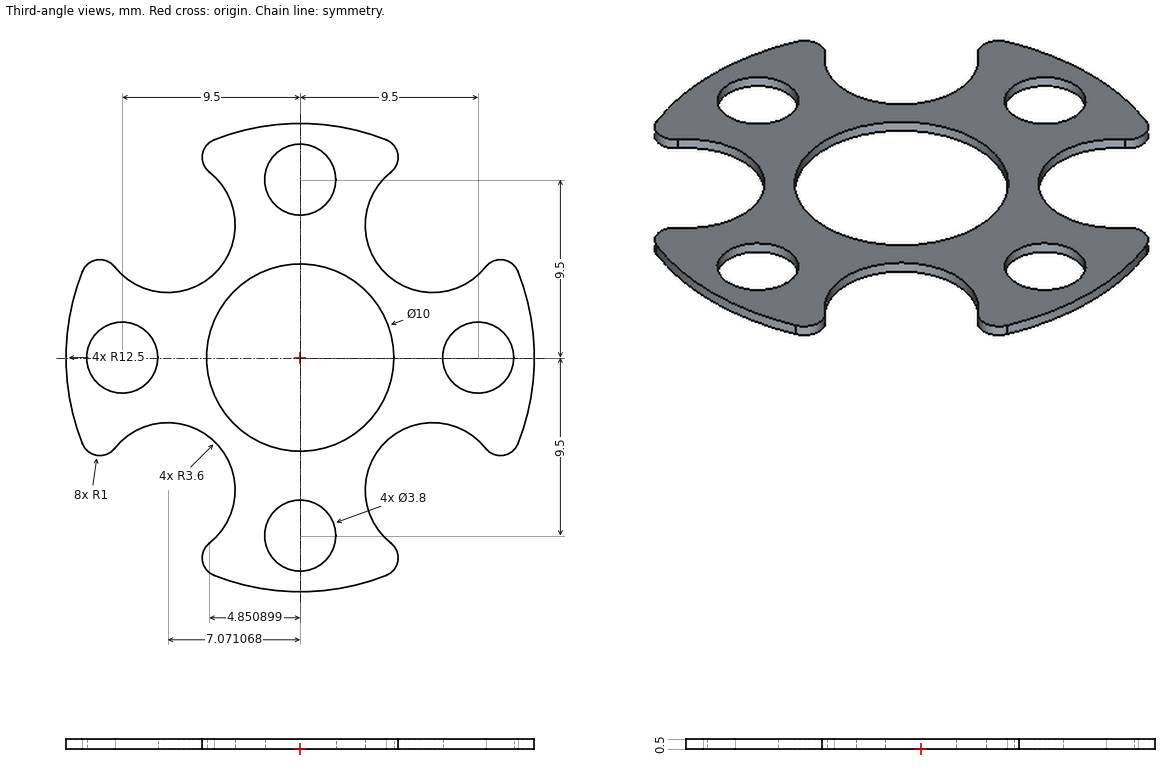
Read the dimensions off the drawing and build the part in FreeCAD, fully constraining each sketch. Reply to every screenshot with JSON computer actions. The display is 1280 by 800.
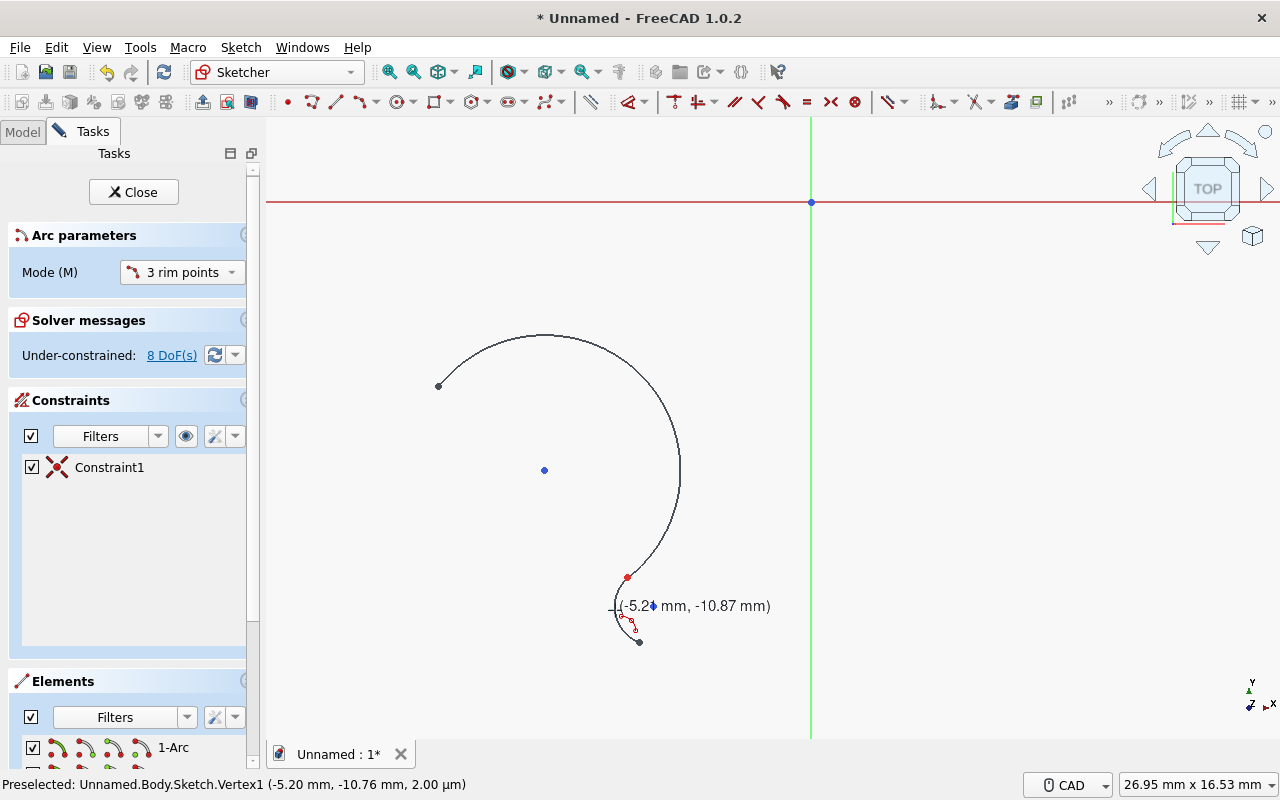
{"action": "left_click", "coordinate": [639, 642]}
{"action": "left_click", "coordinate": [984, 639]}
{"action": "left_click", "coordinate": [776, 671]}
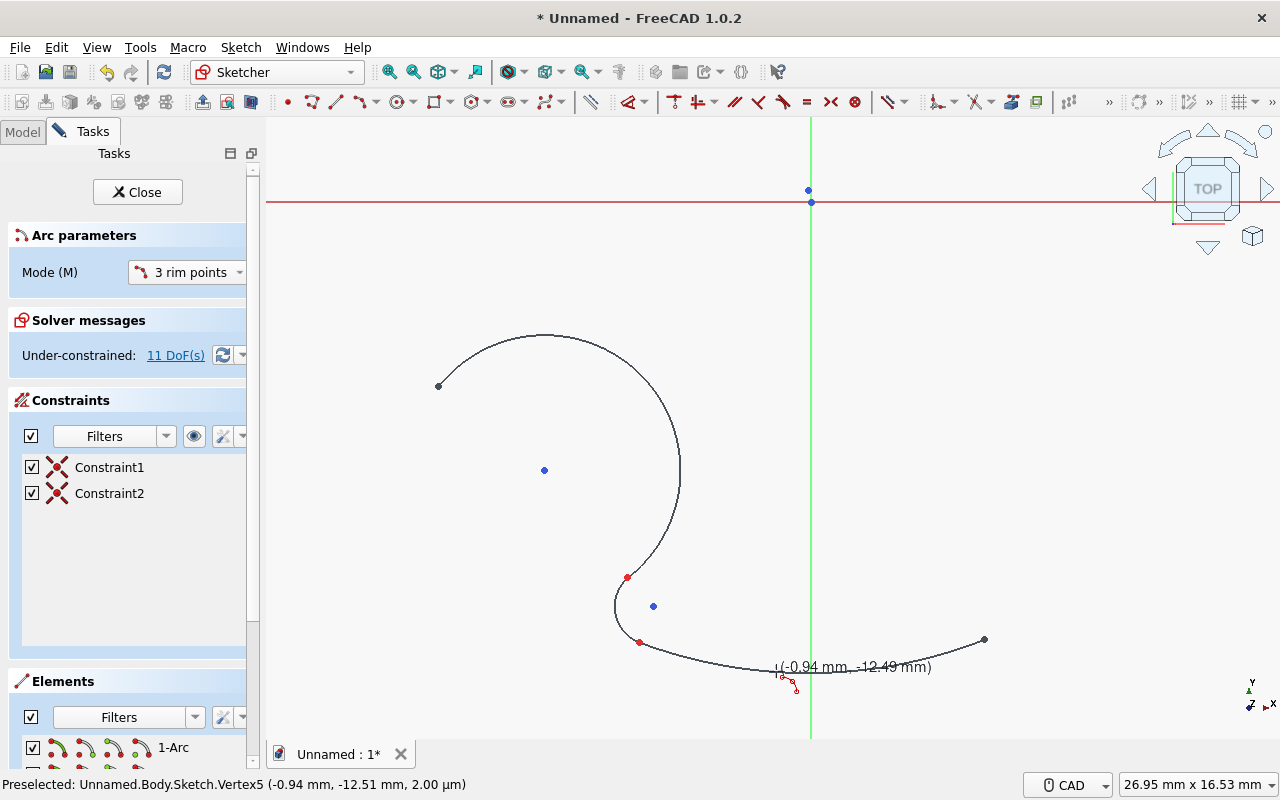
{"action": "left_click", "coordinate": [984, 640]}
{"action": "left_click", "coordinate": [994, 575]}
{"action": "left_click", "coordinate": [1008, 610]}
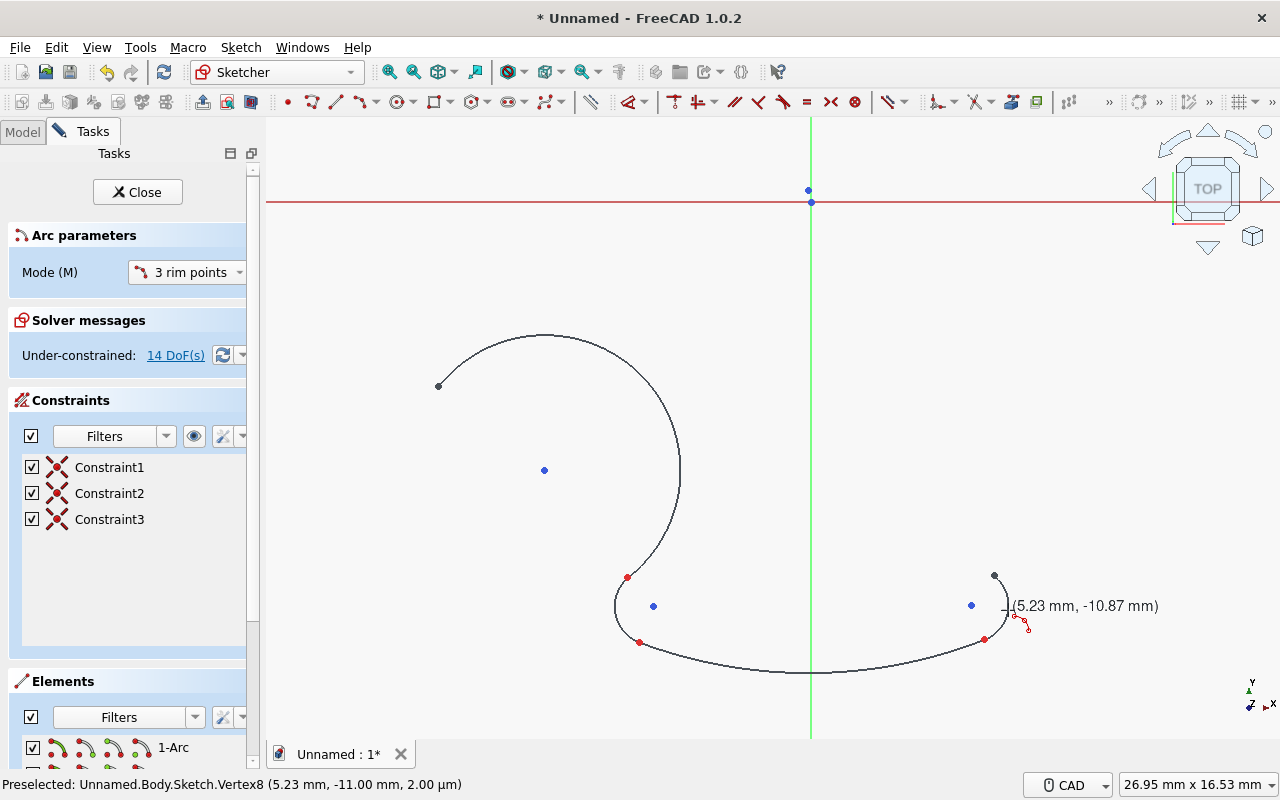
{"action": "left_click", "coordinate": [994, 576]}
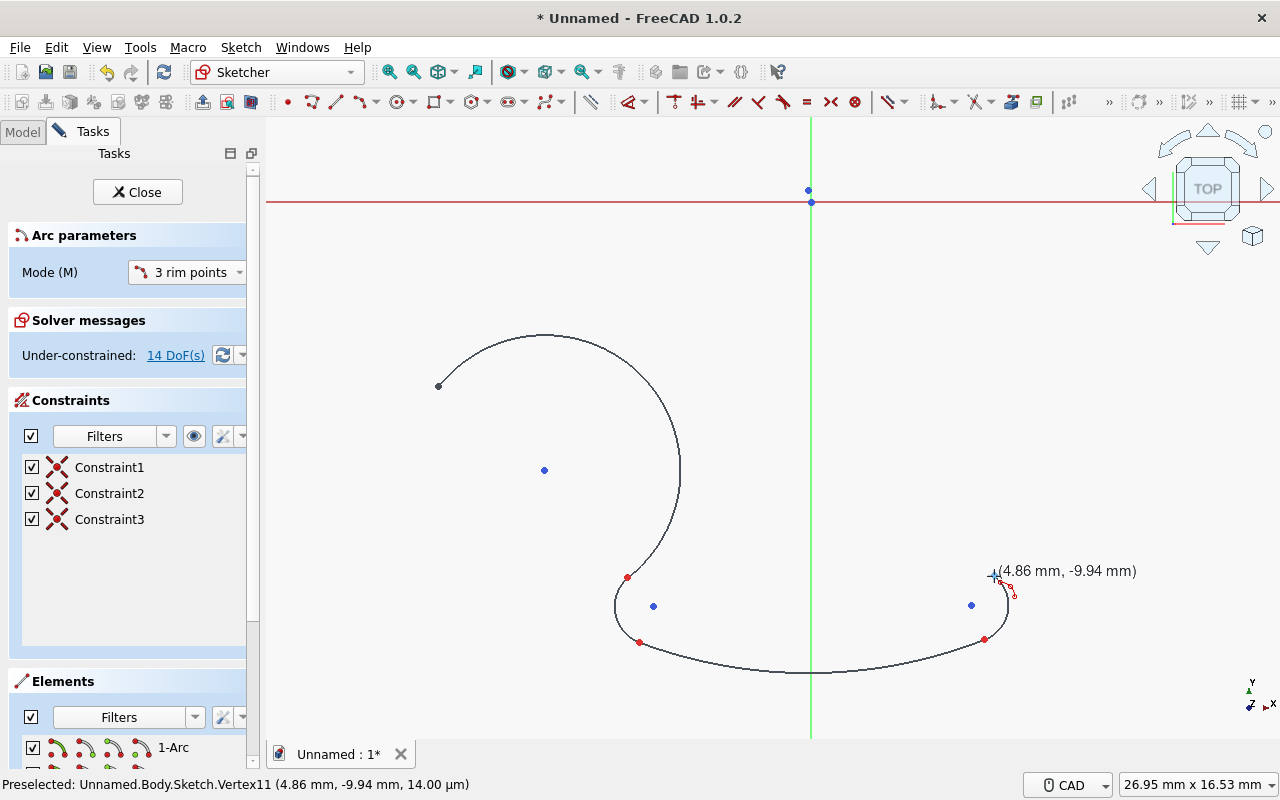
{"action": "scroll", "coordinate": [617, 612], "scroll_direction": "down", "scroll_amount": 4}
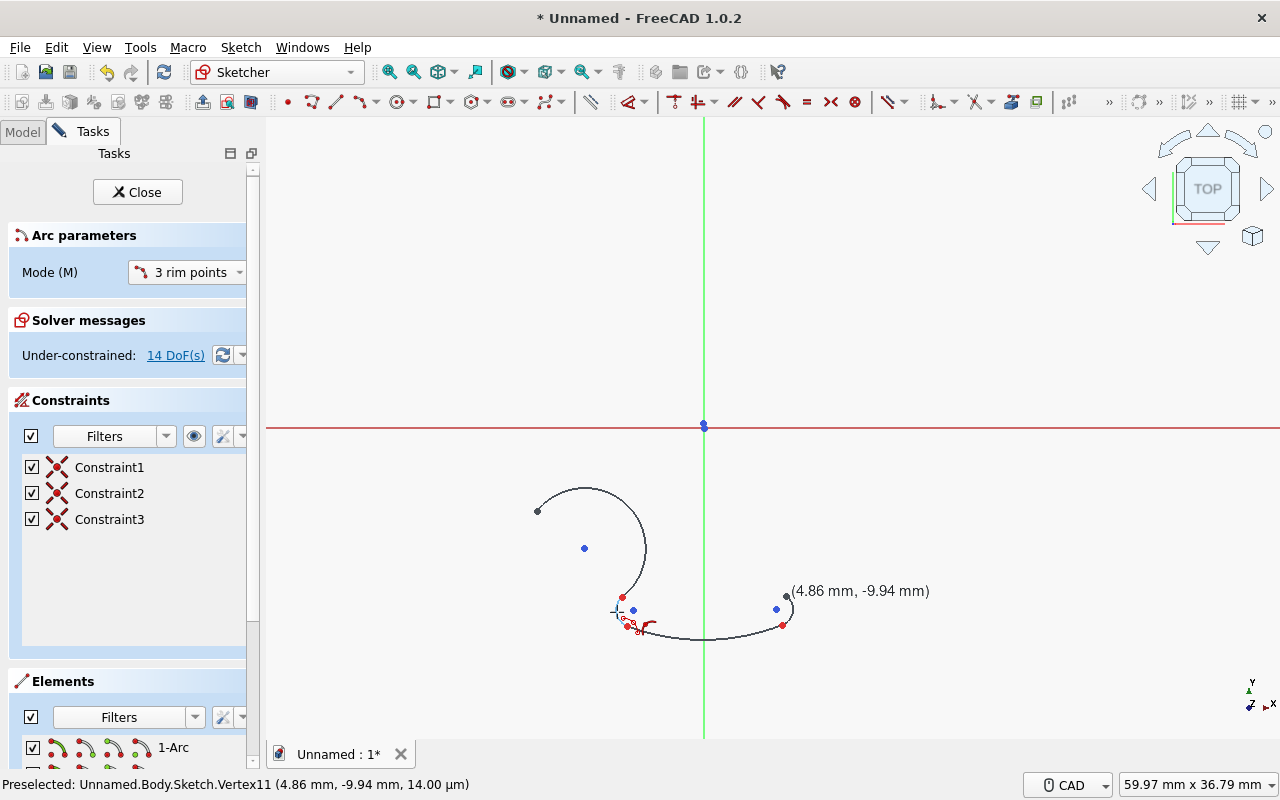
{"action": "left_click", "coordinate": [872, 510]}
{"action": "left_click", "coordinate": [781, 505]}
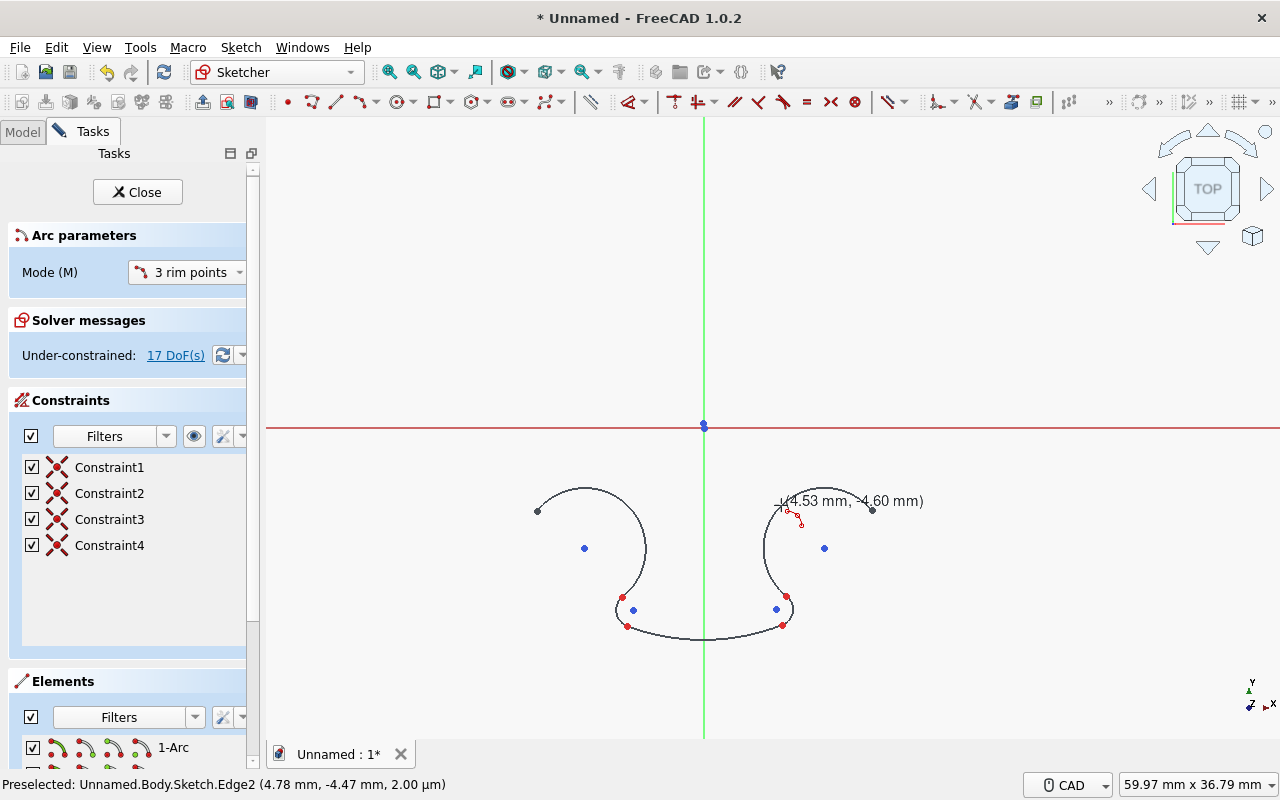
{"action": "left_click", "coordinate": [872, 511]}
{"action": "left_click", "coordinate": [901, 506]}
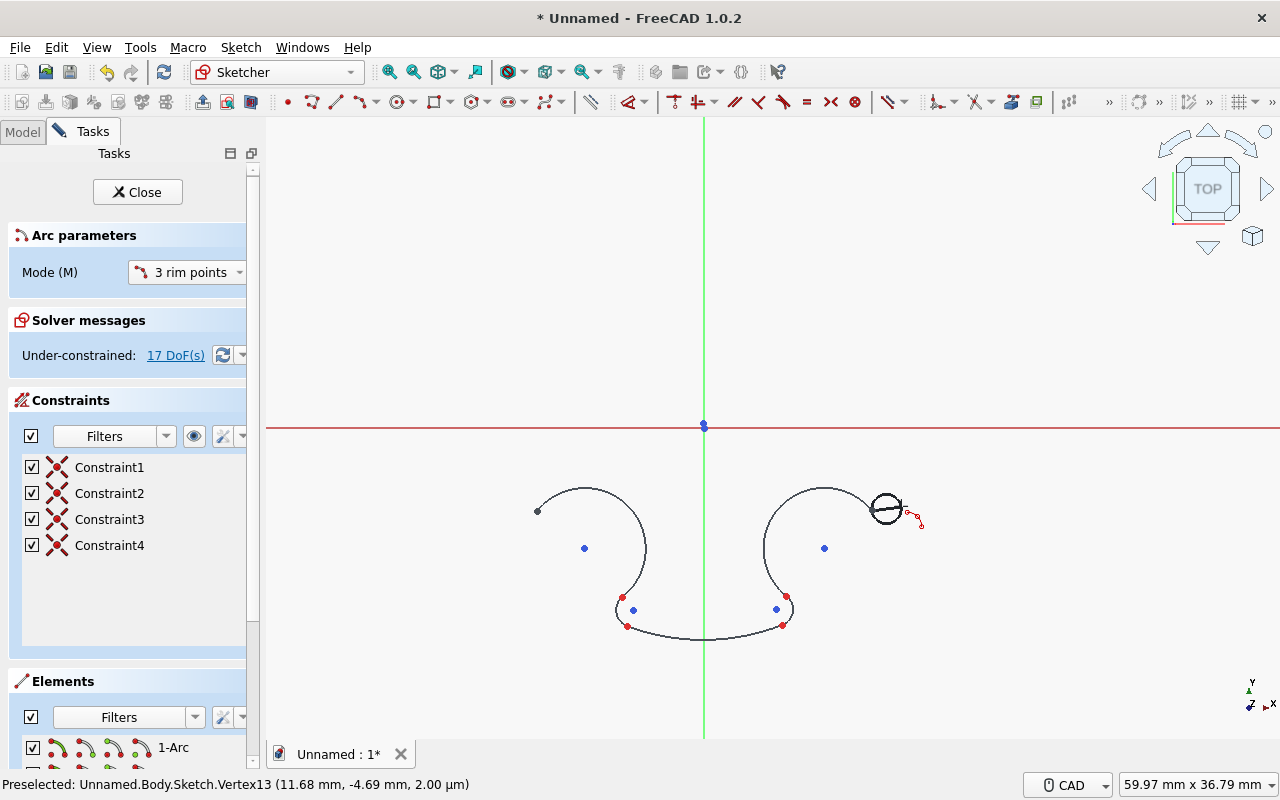
{"action": "scroll", "coordinate": [888, 517], "scroll_direction": "up", "scroll_amount": 4}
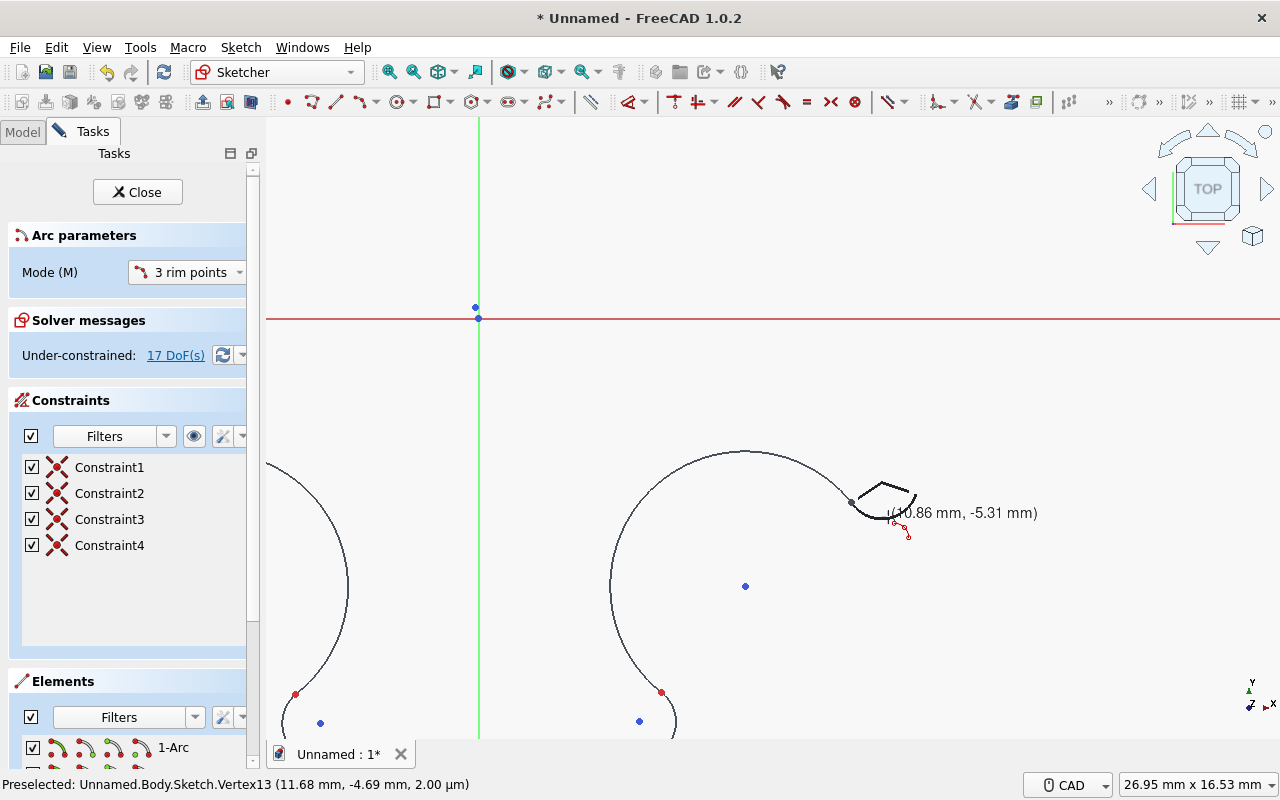
{"action": "left_click", "coordinate": [886, 515]}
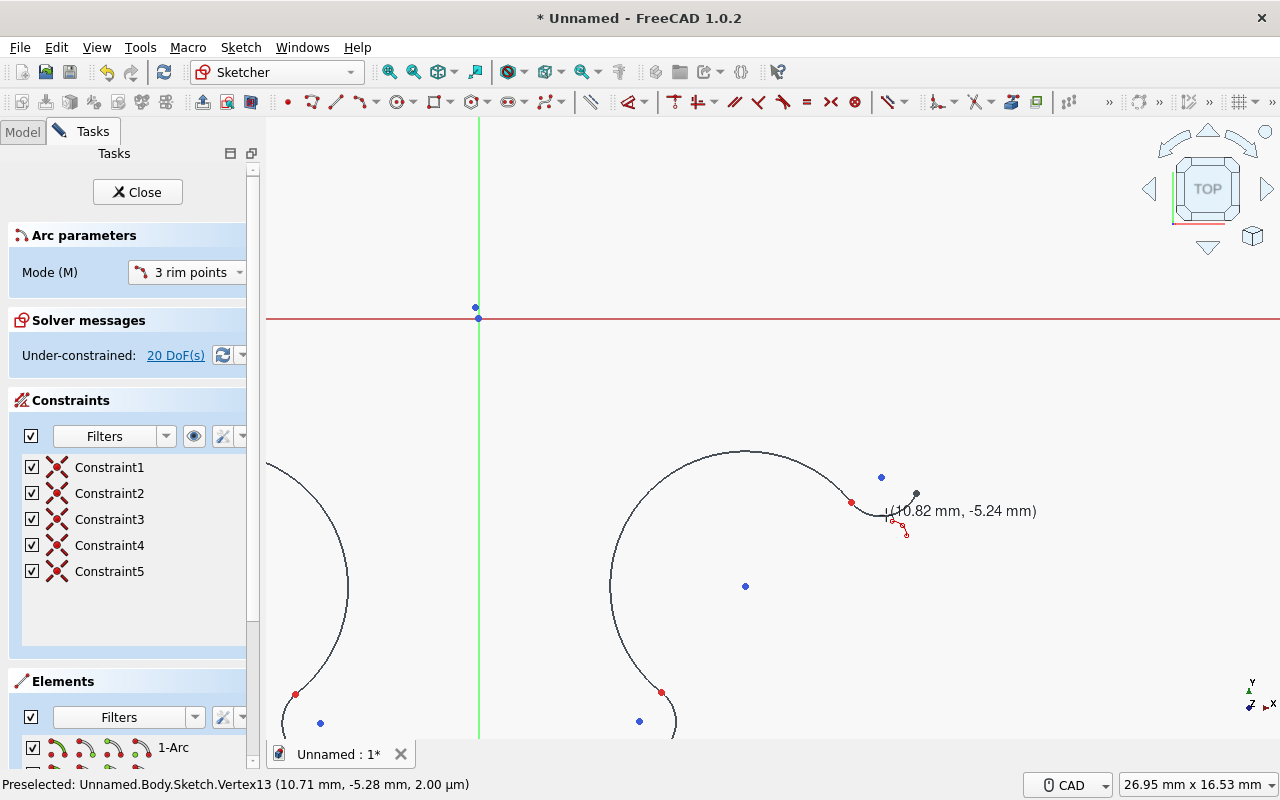
{"action": "left_click", "coordinate": [916, 494]}
{"action": "left_click", "coordinate": [916, 145]}
{"action": "left_click", "coordinate": [948, 354]}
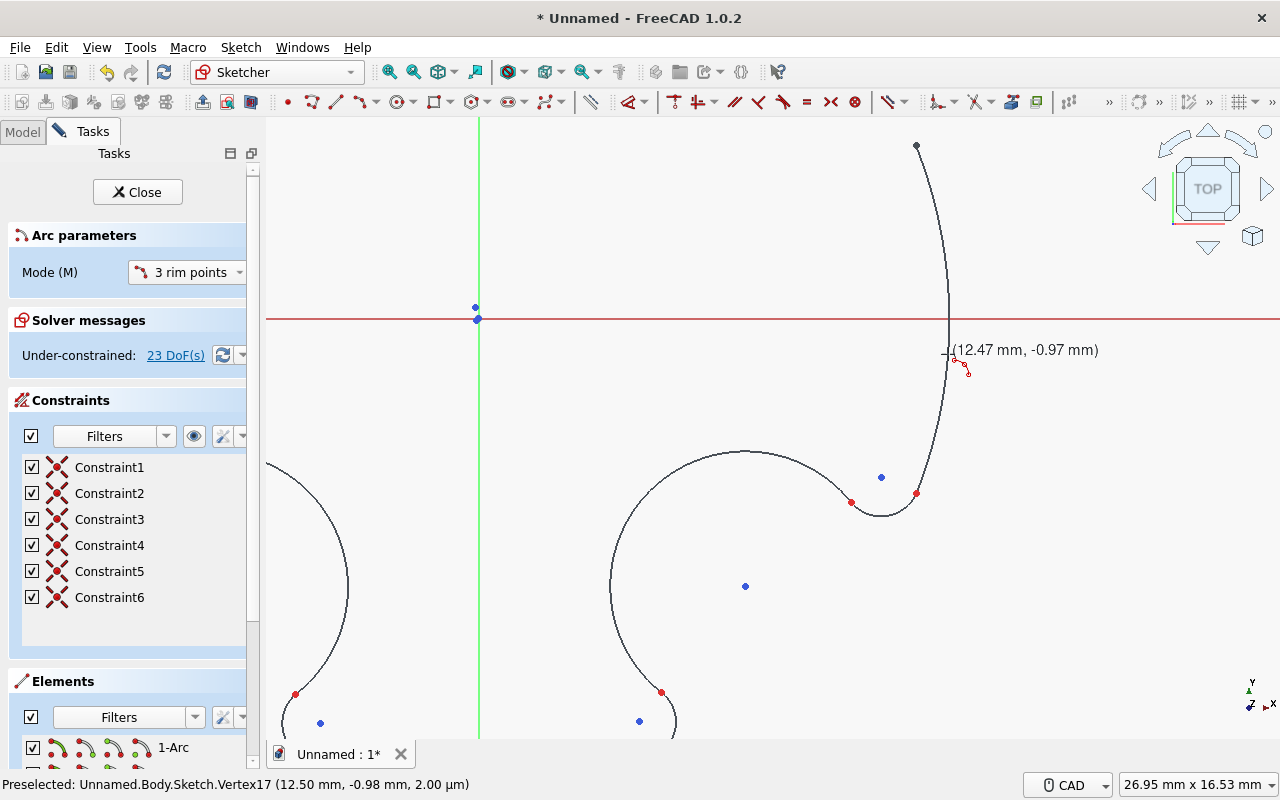
{"action": "left_click", "coordinate": [916, 146]}